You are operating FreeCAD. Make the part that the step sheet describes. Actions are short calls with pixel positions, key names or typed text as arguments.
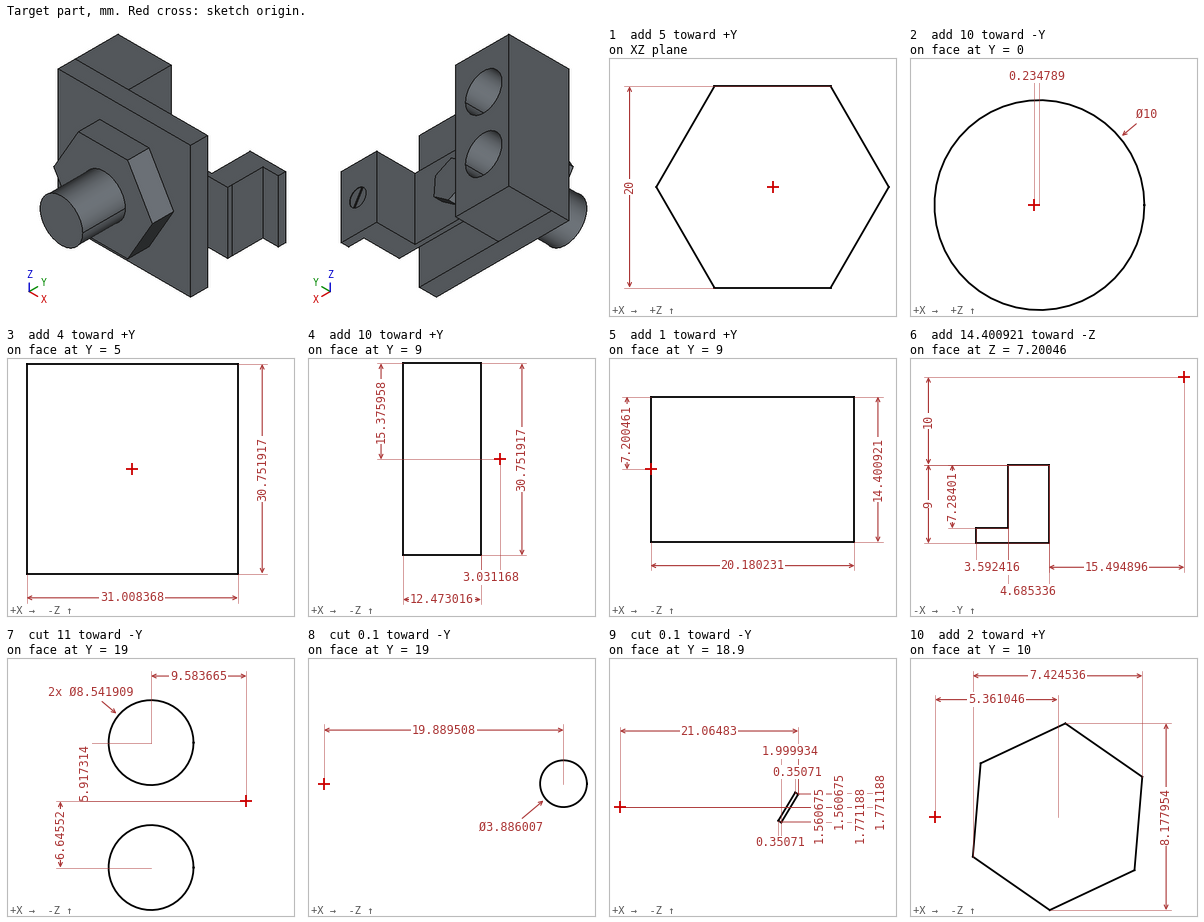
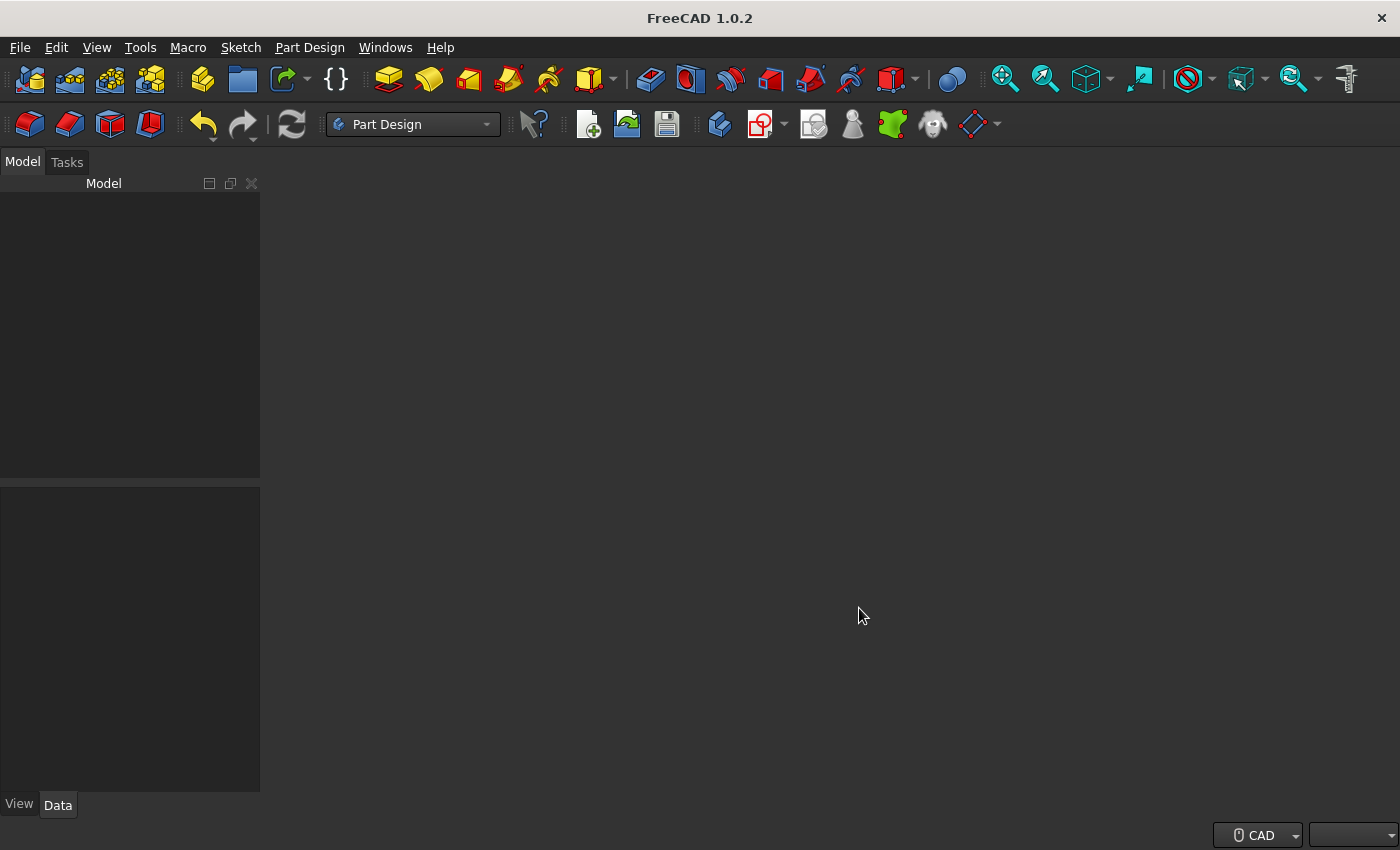
click(588, 124)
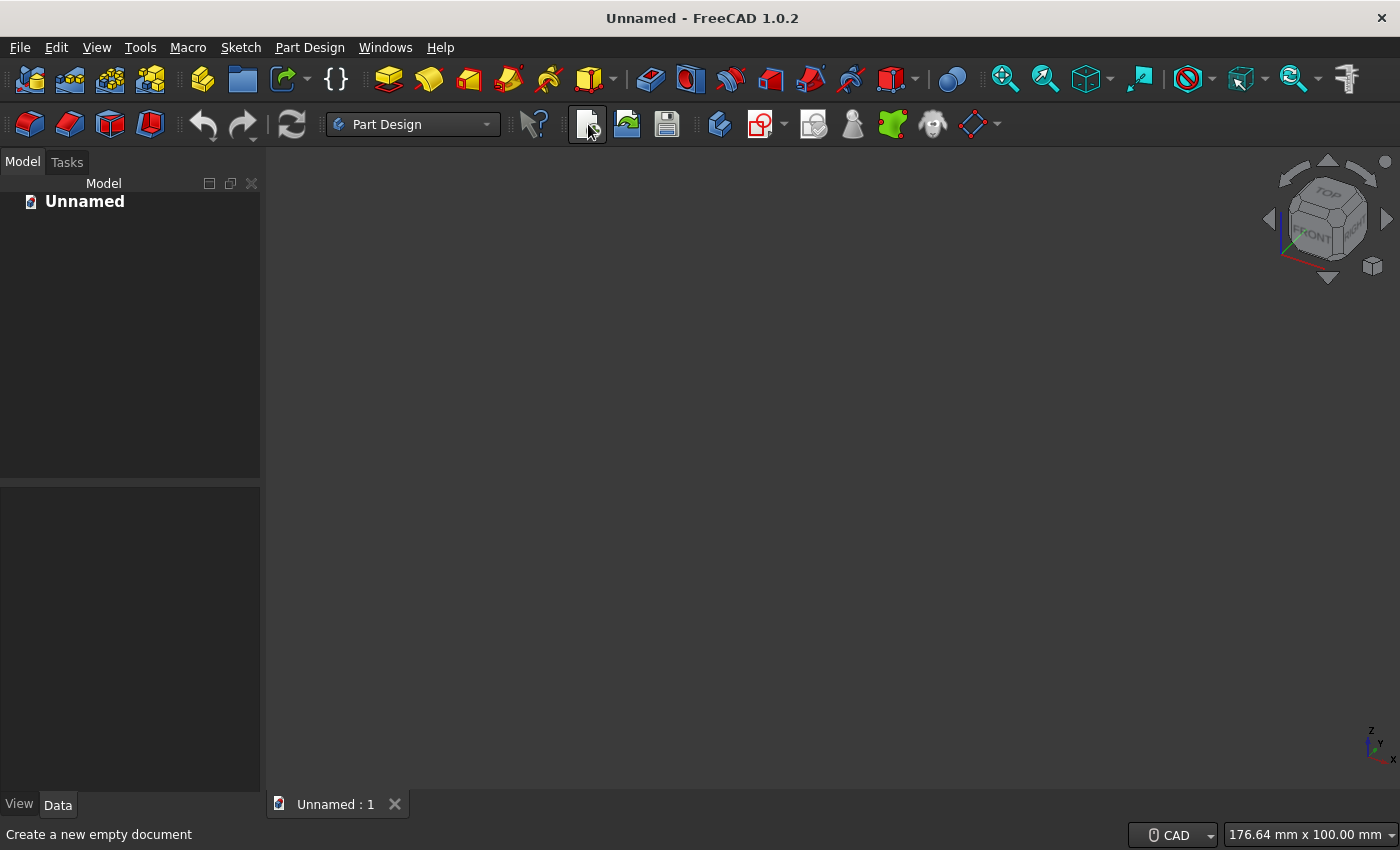
click(760, 124)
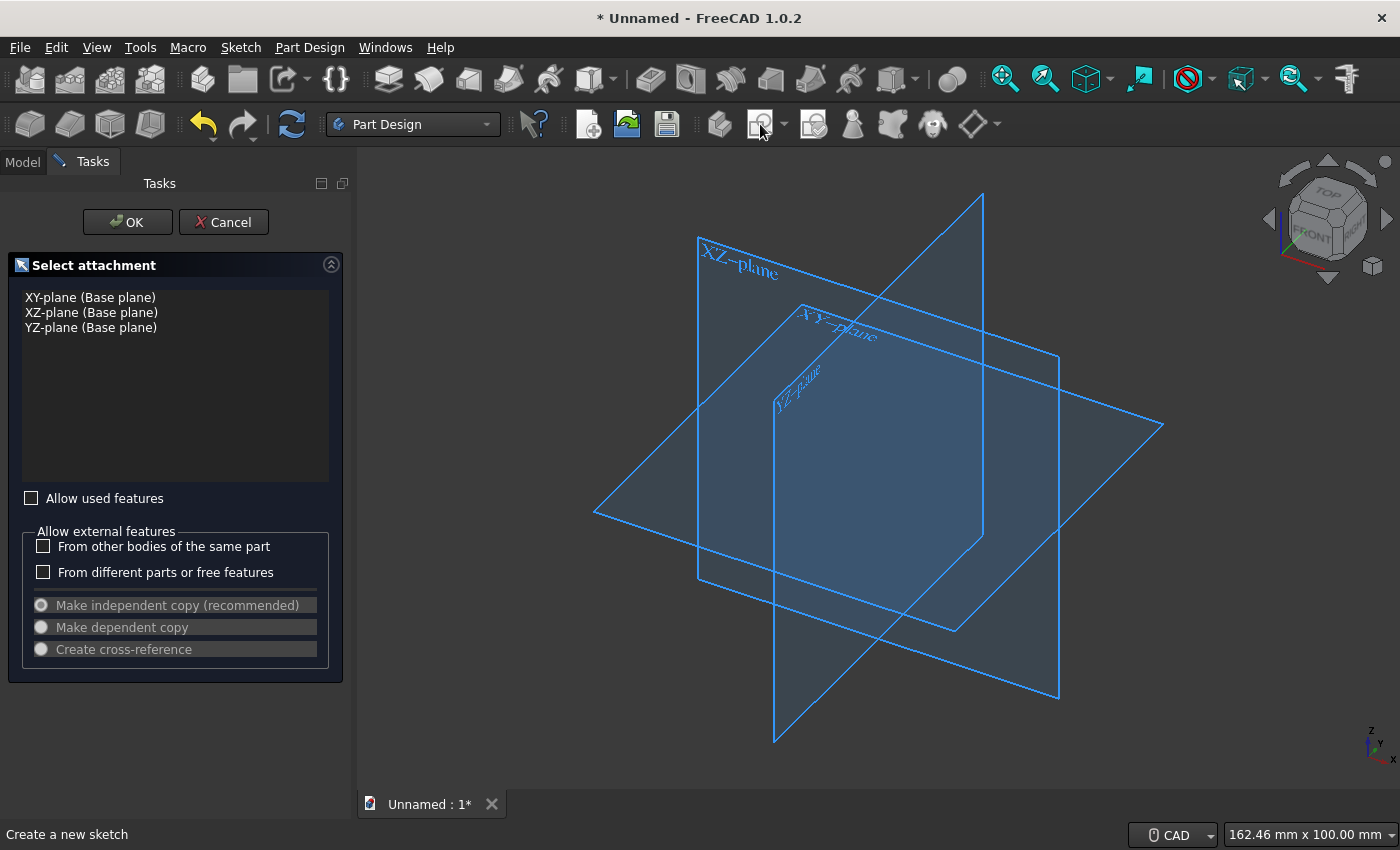
click(82, 312)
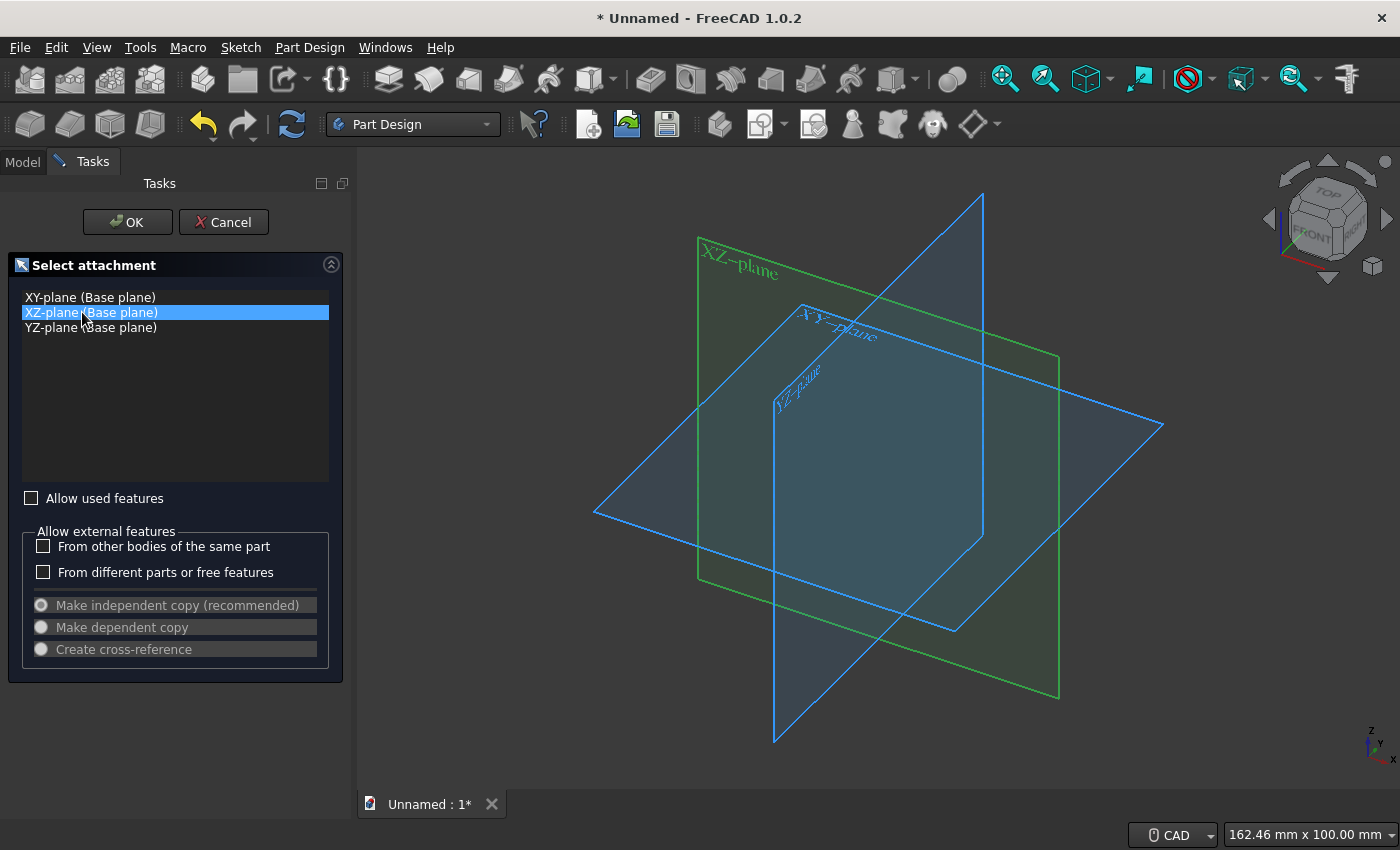
click(128, 222)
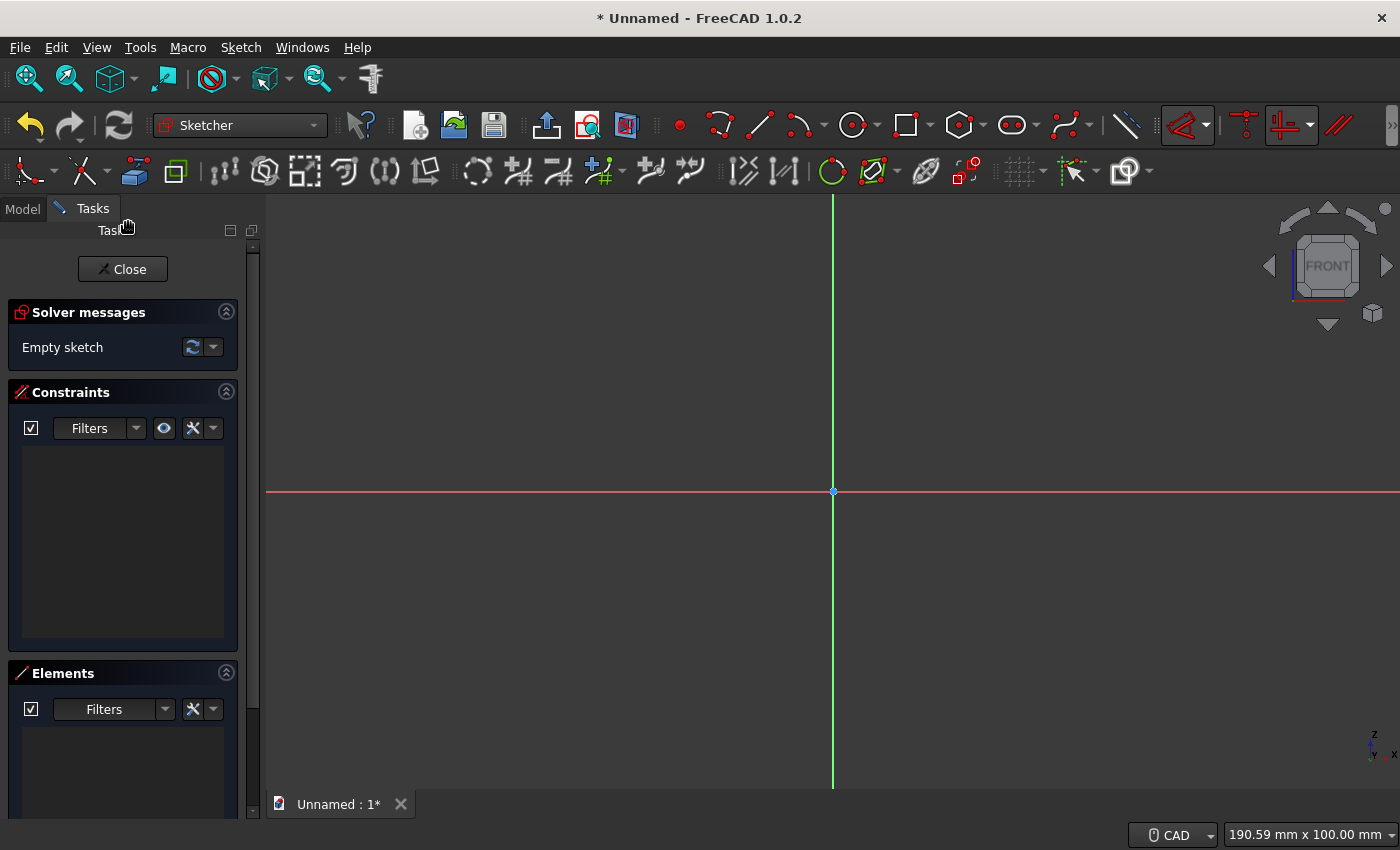
scroll(863, 492, up, 6)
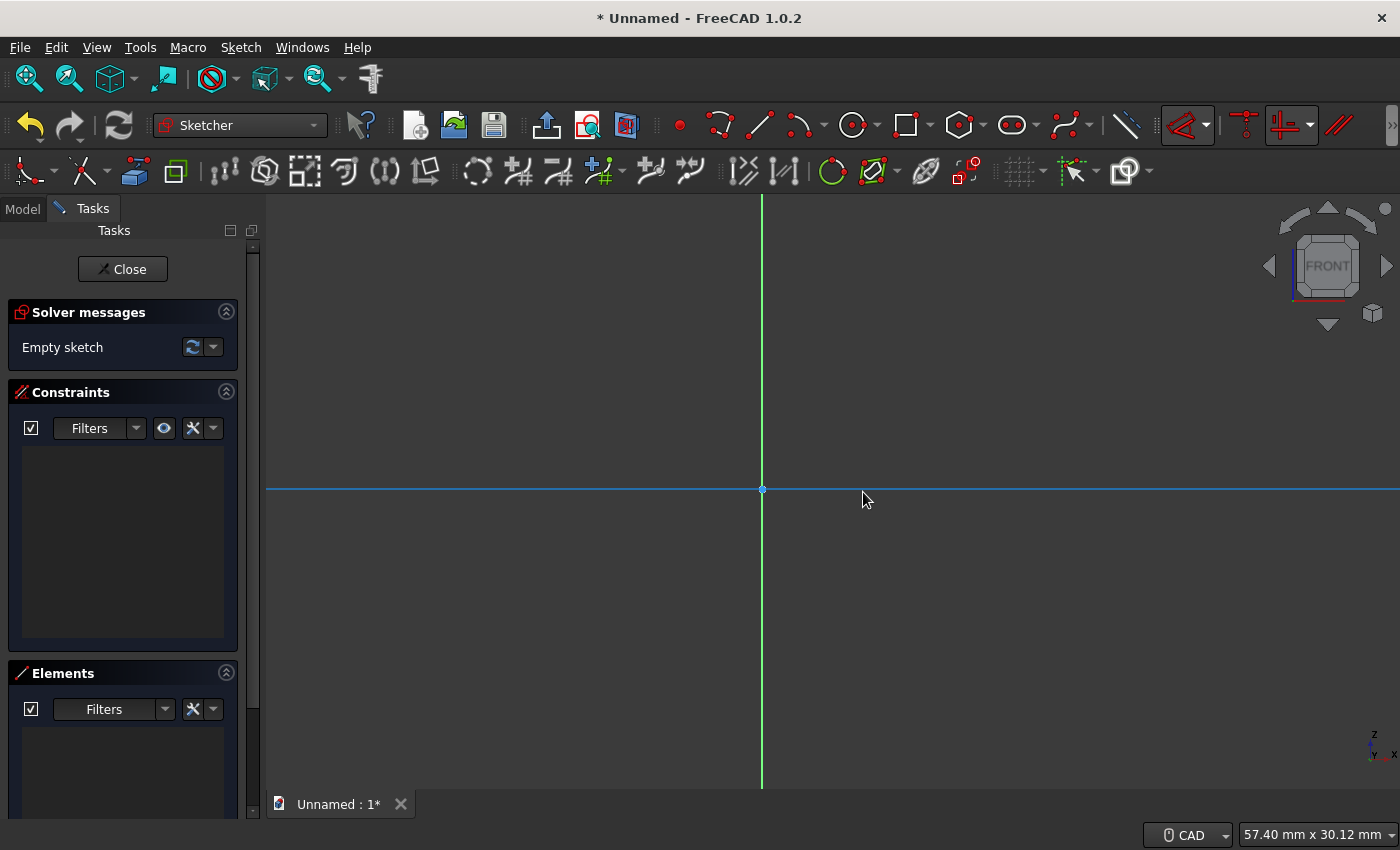
click(960, 126)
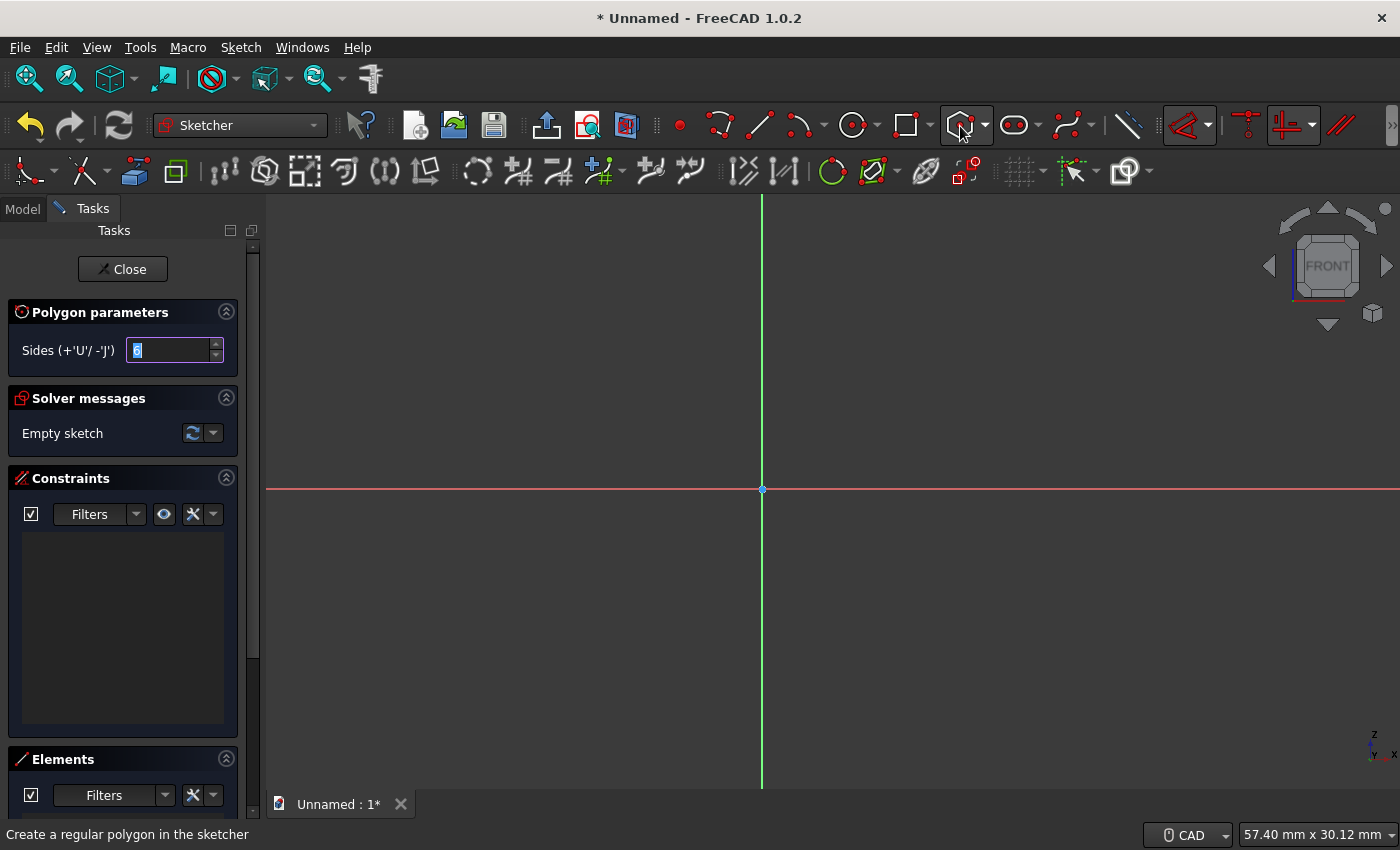
click(762, 489)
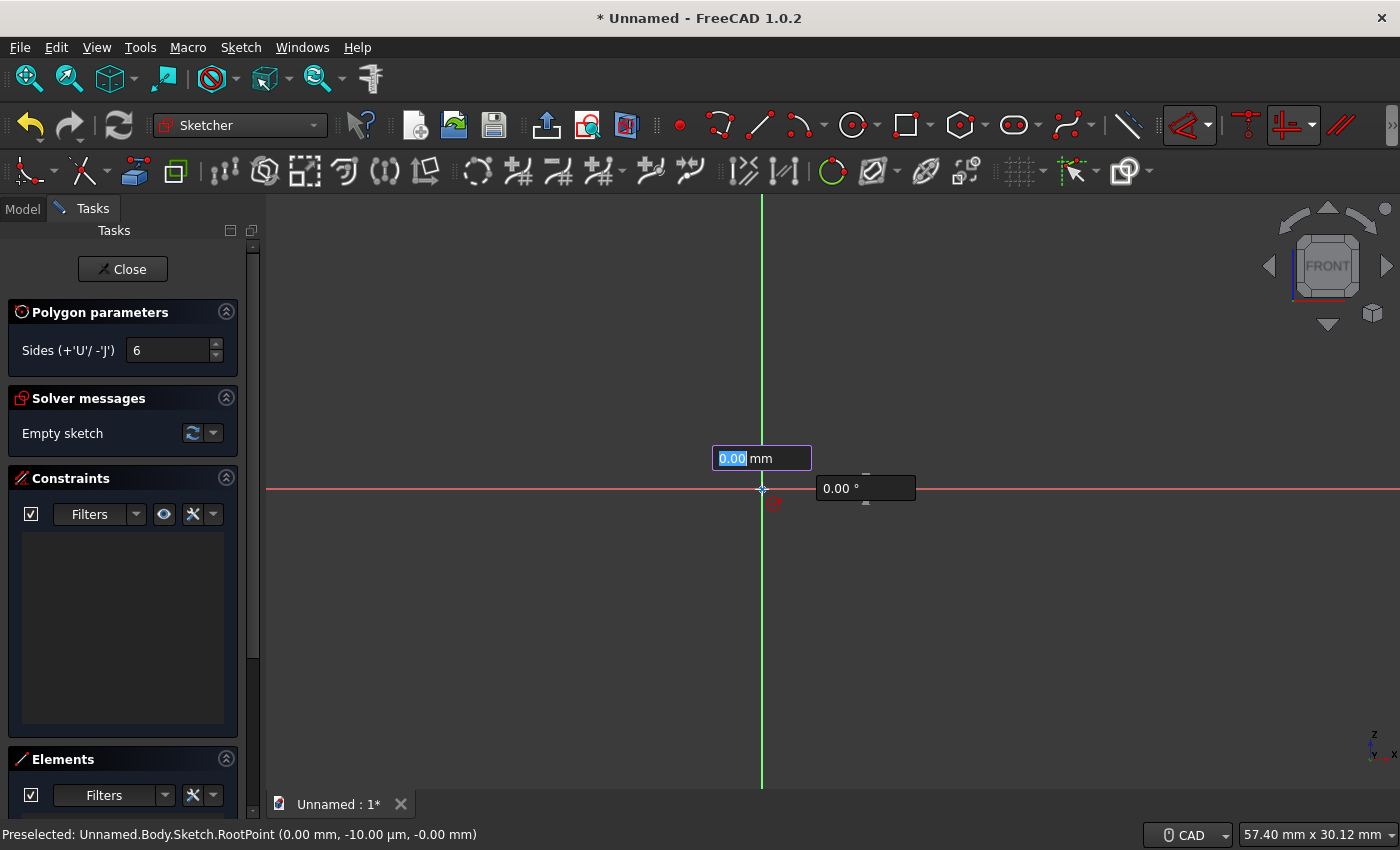
click(534, 489)
right_click(534, 489)